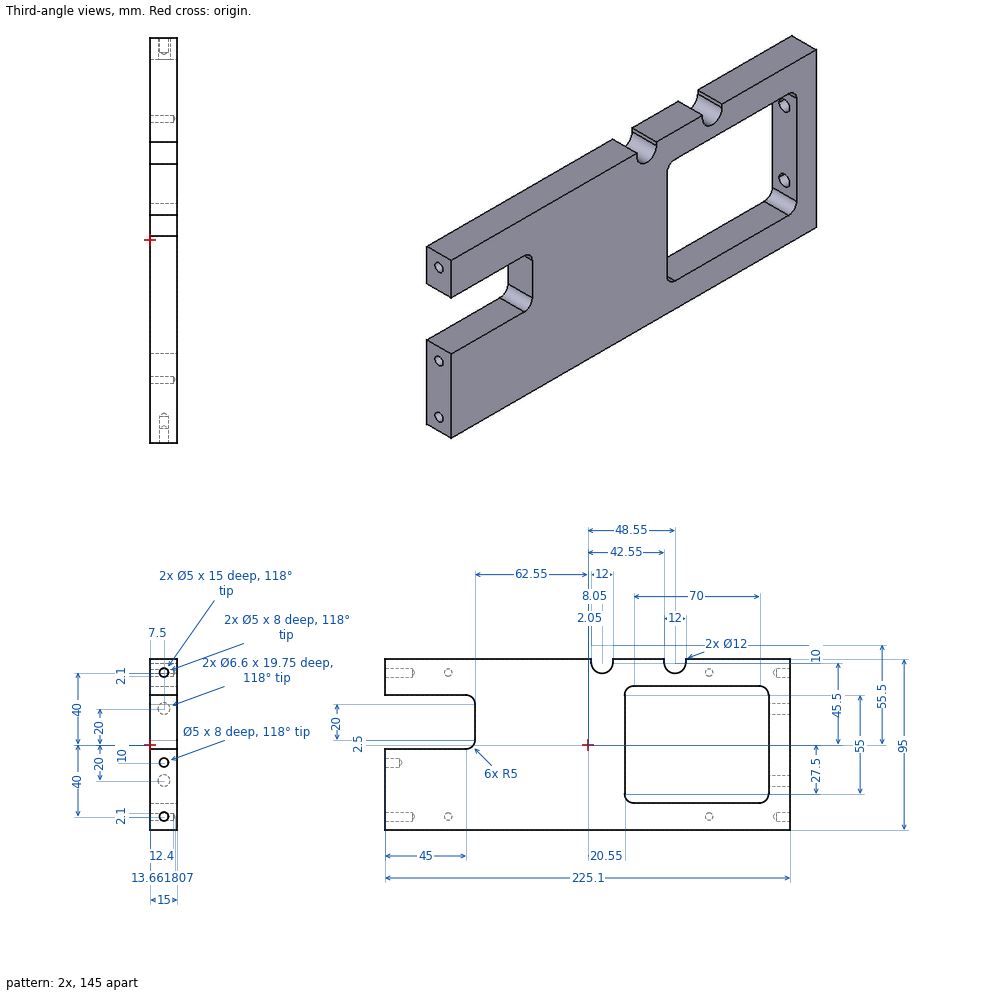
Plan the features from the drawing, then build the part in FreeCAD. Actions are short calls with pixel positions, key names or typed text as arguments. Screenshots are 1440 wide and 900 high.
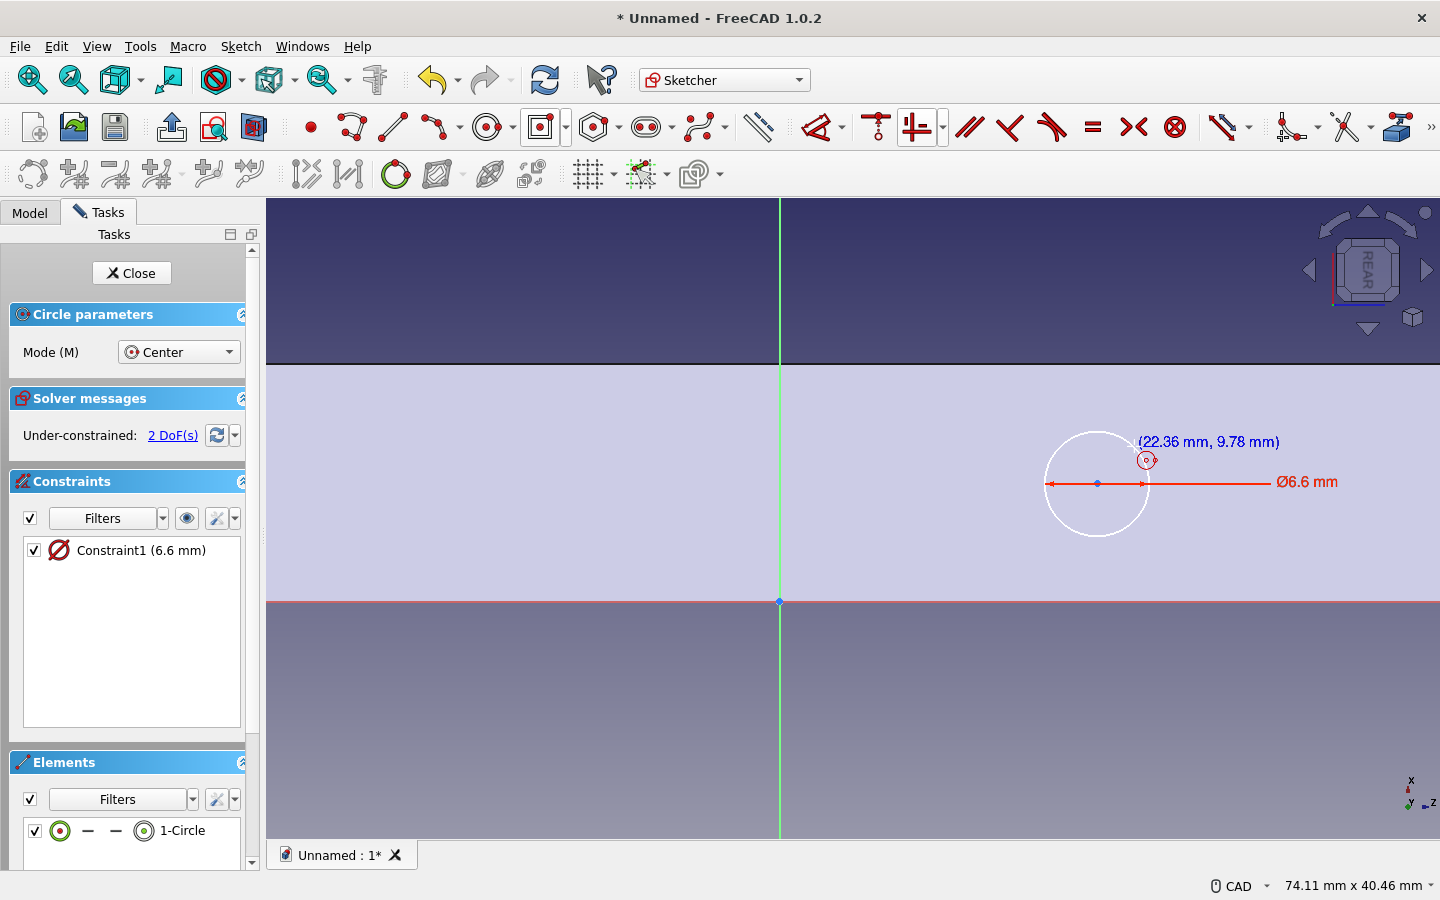
click(463, 483)
move(500, 446)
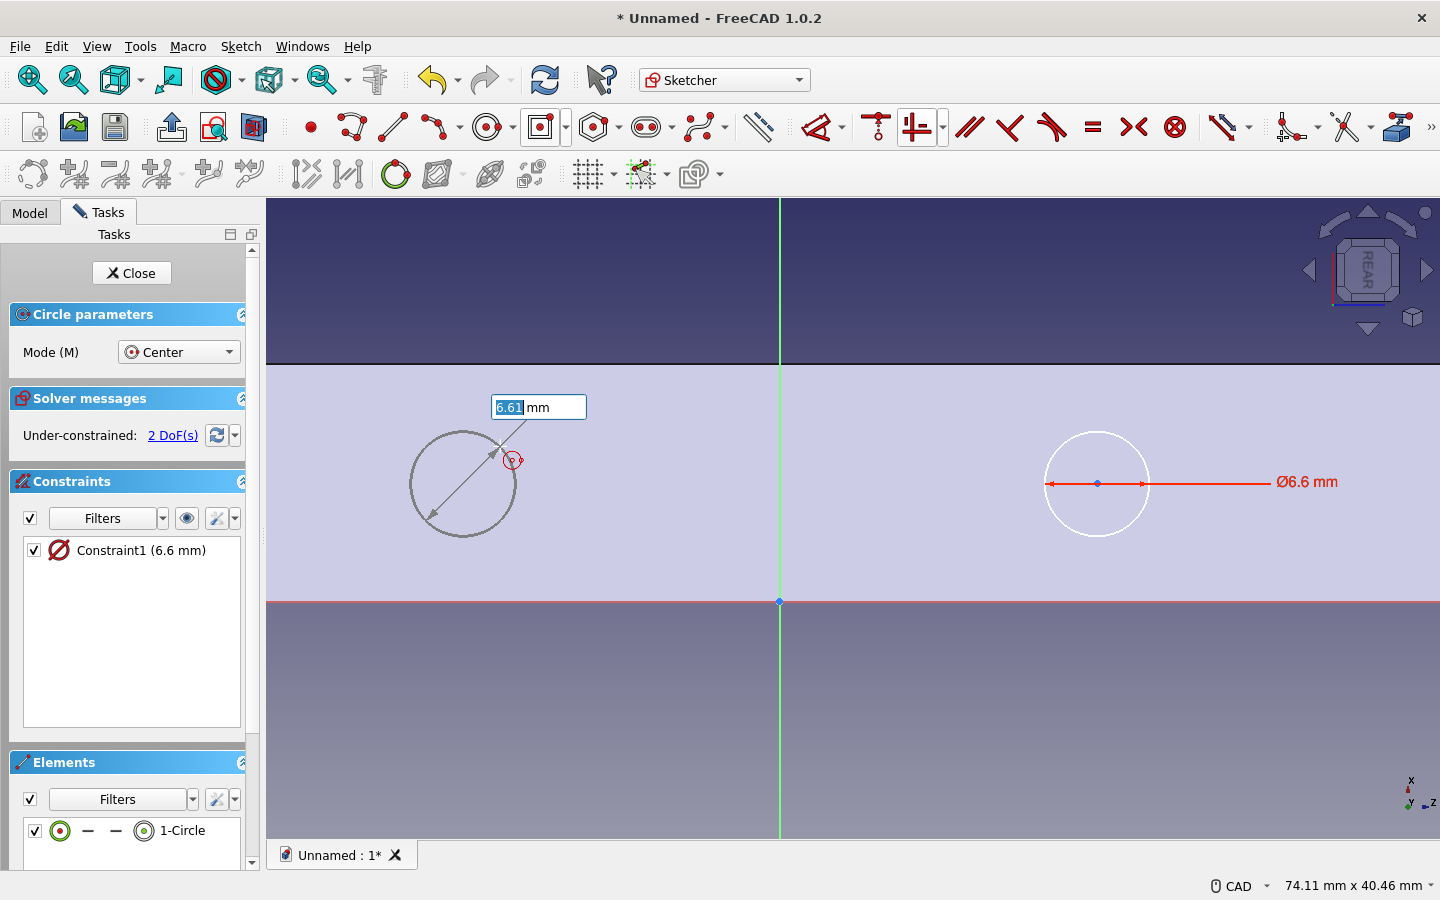
text(6.6)
key(Return)
key(Escape)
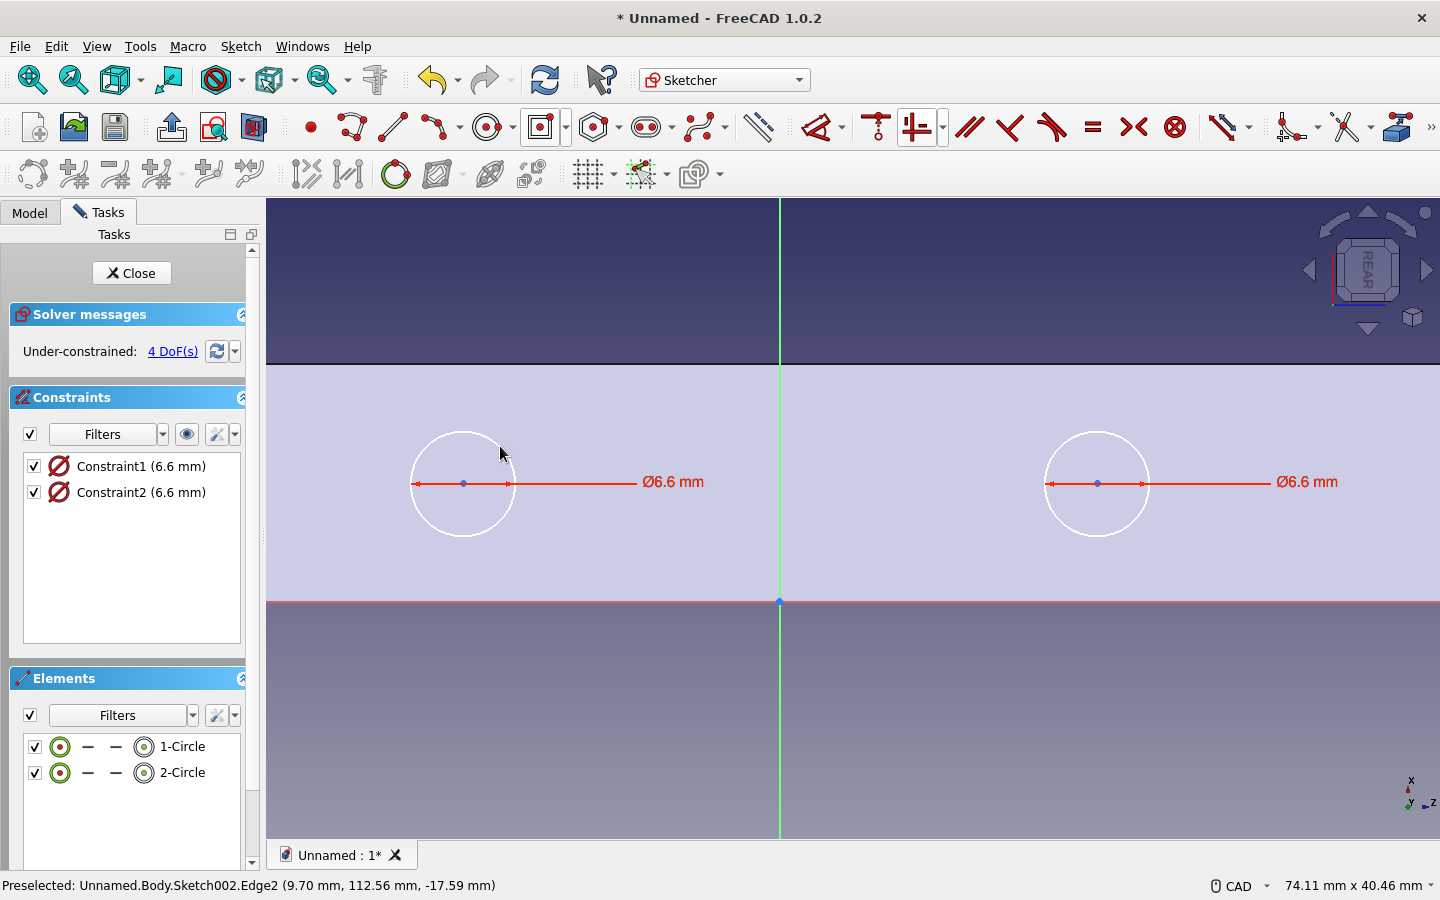
click(1097, 484)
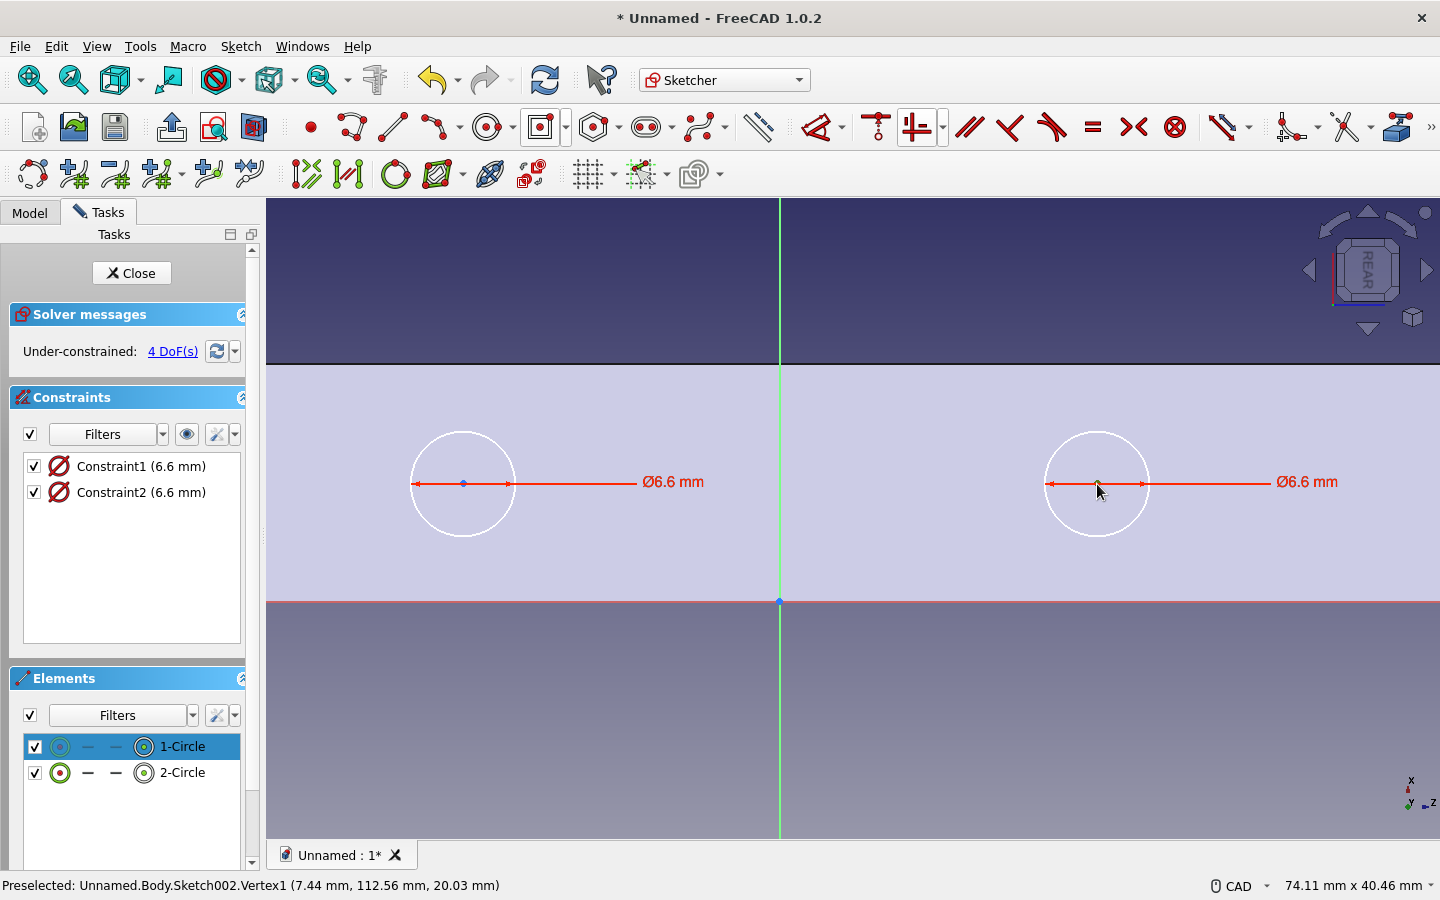
click(463, 484)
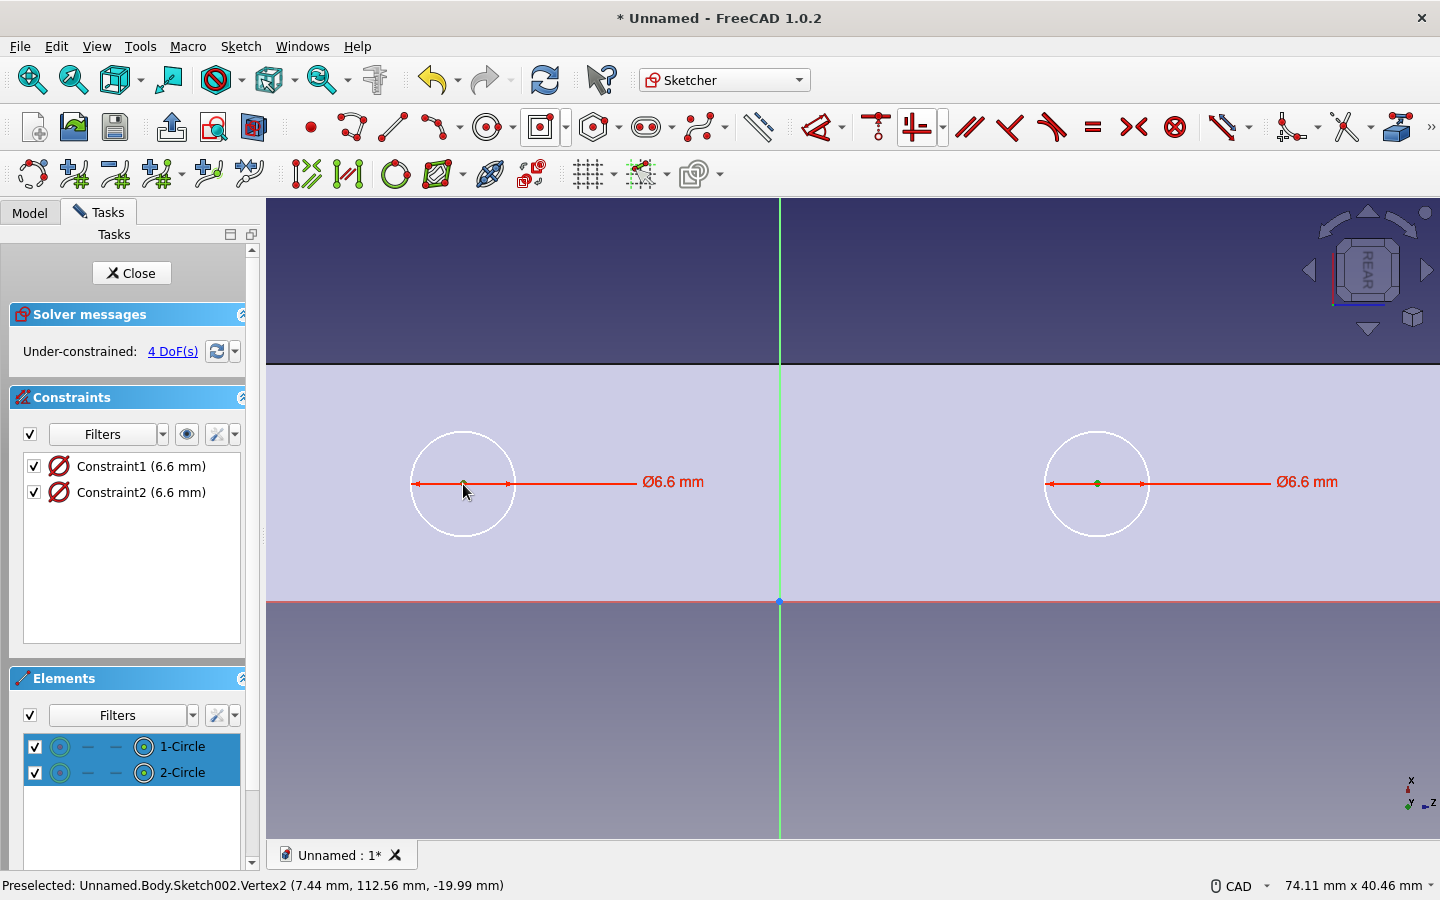
click(942, 128)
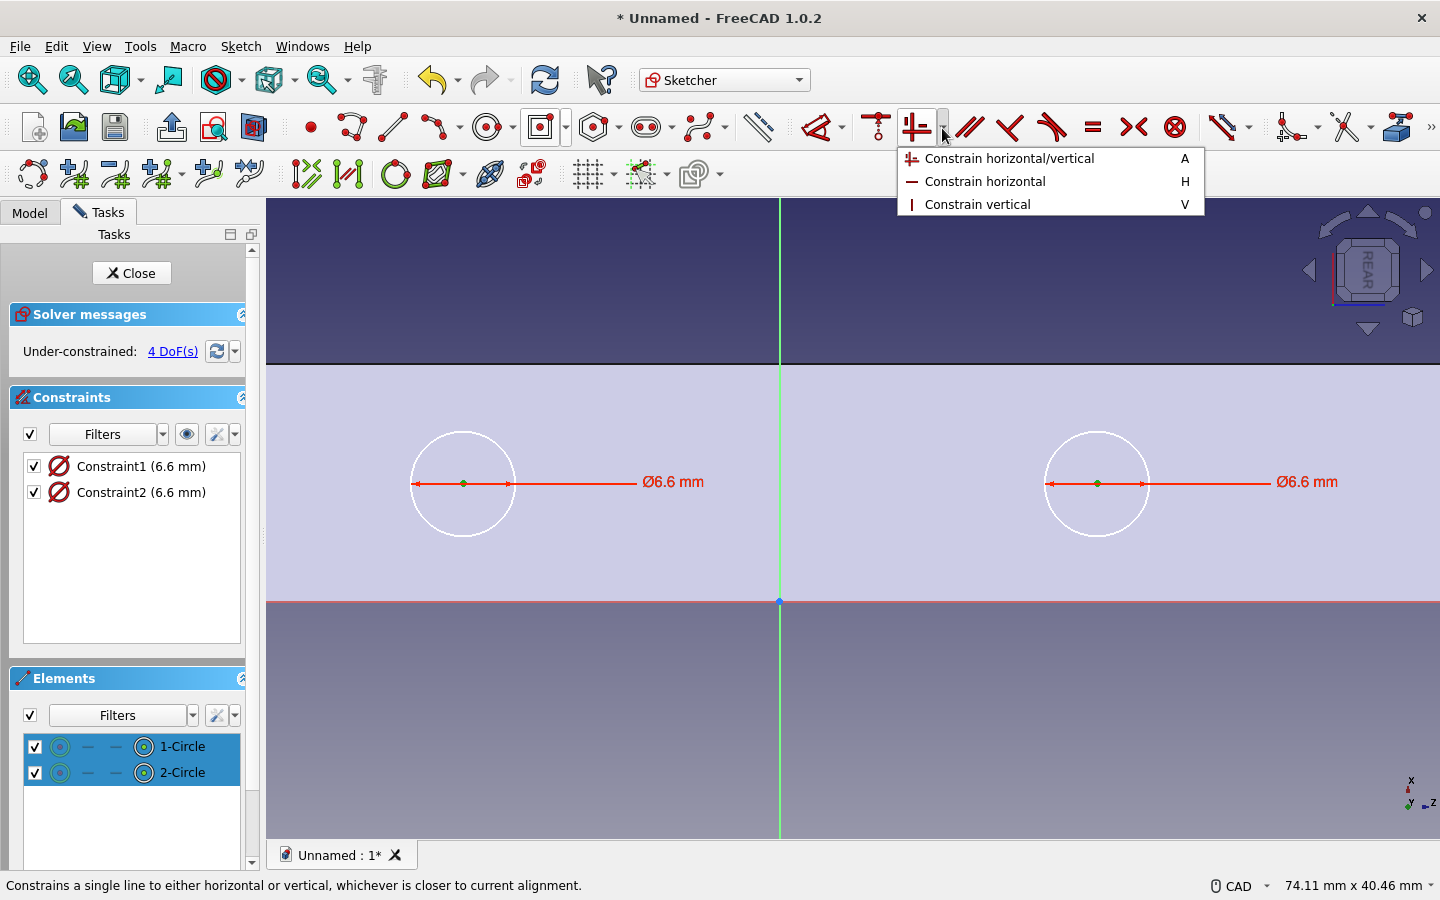
click(1051, 182)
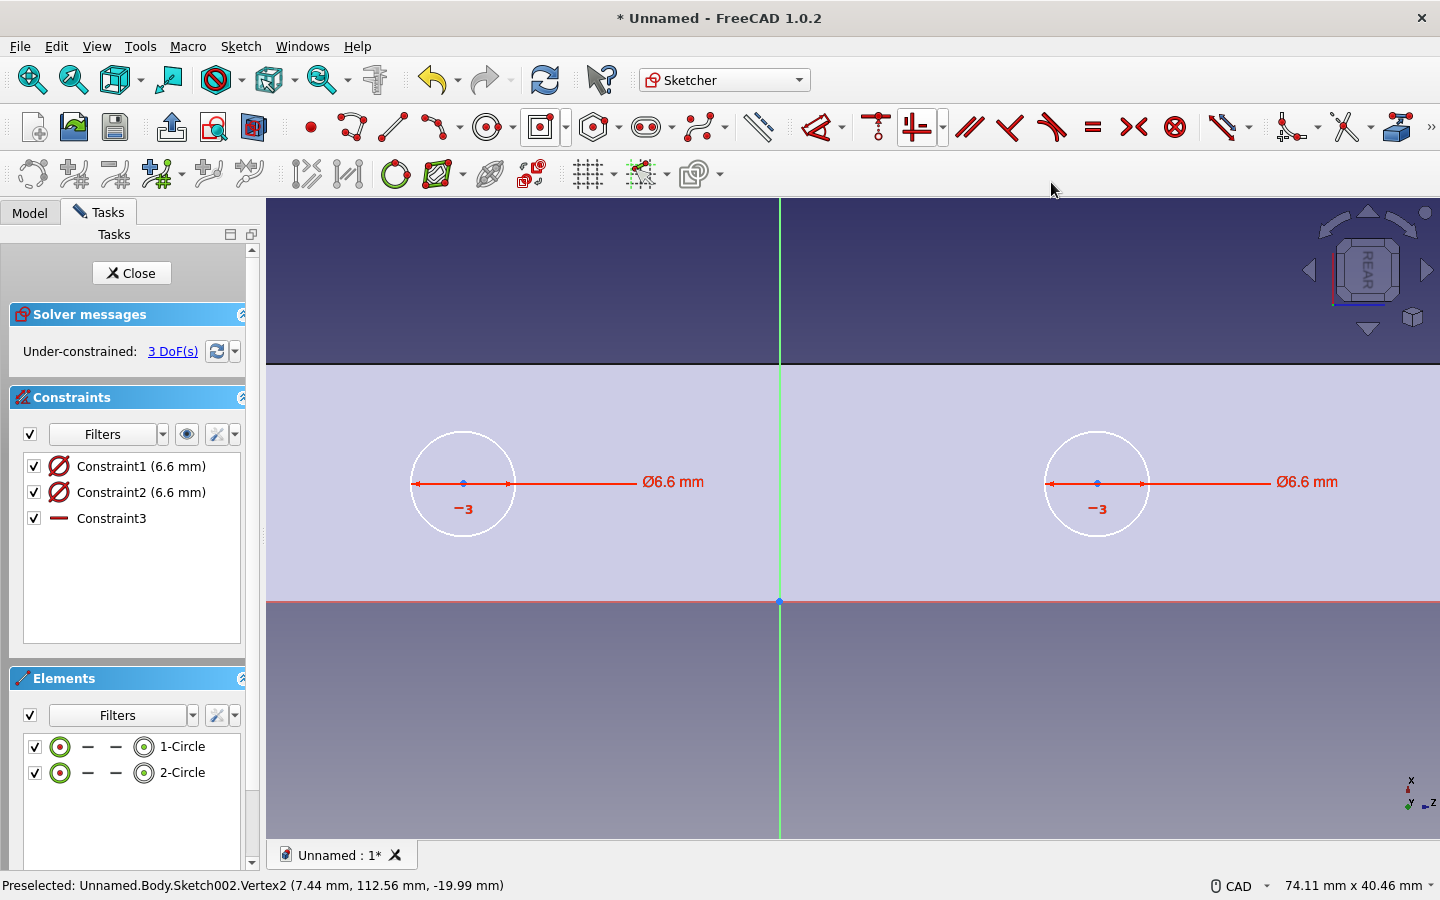
click(816, 128)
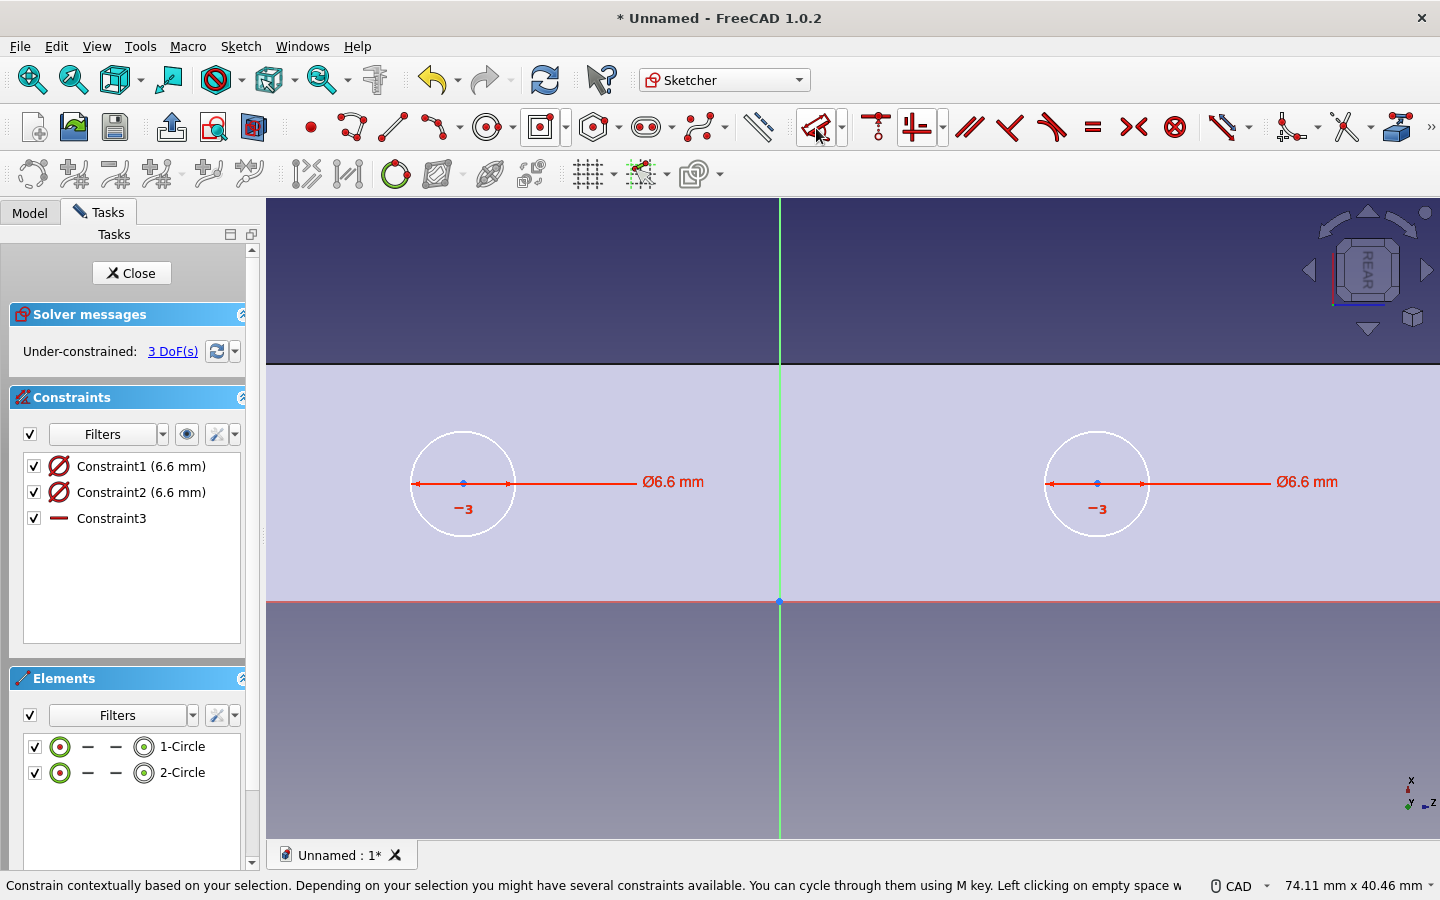
click(1097, 484)
click(938, 636)